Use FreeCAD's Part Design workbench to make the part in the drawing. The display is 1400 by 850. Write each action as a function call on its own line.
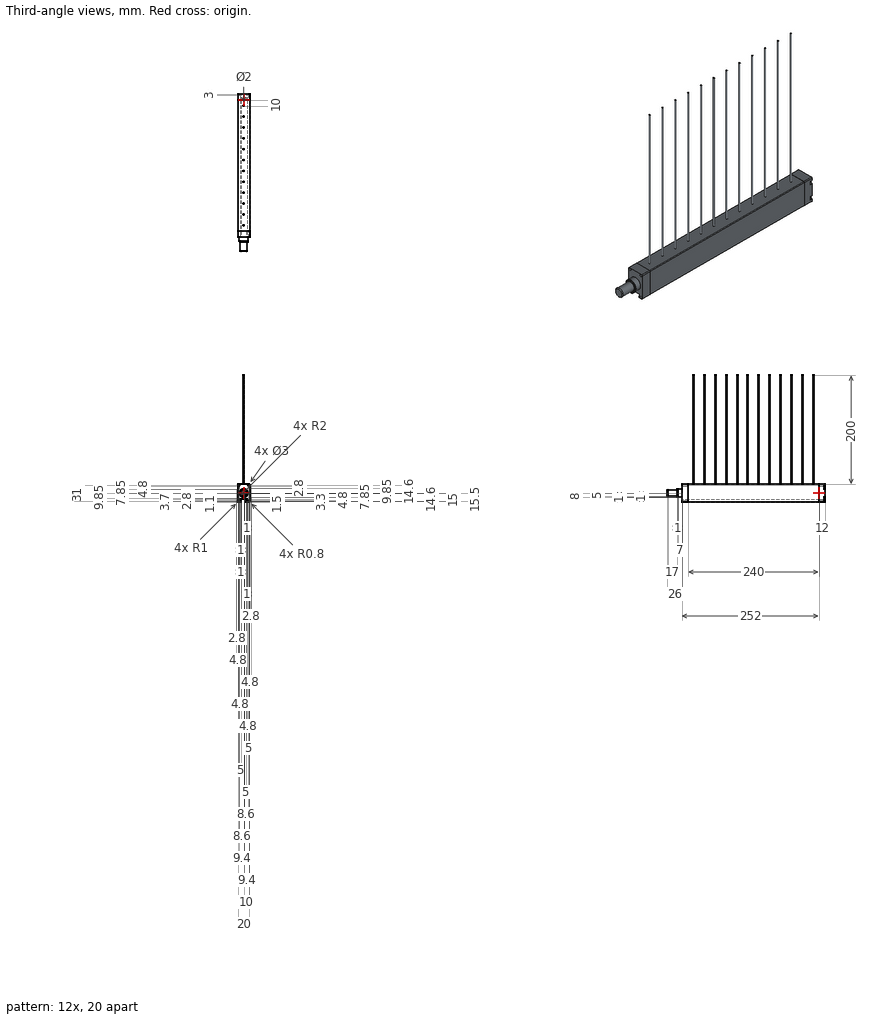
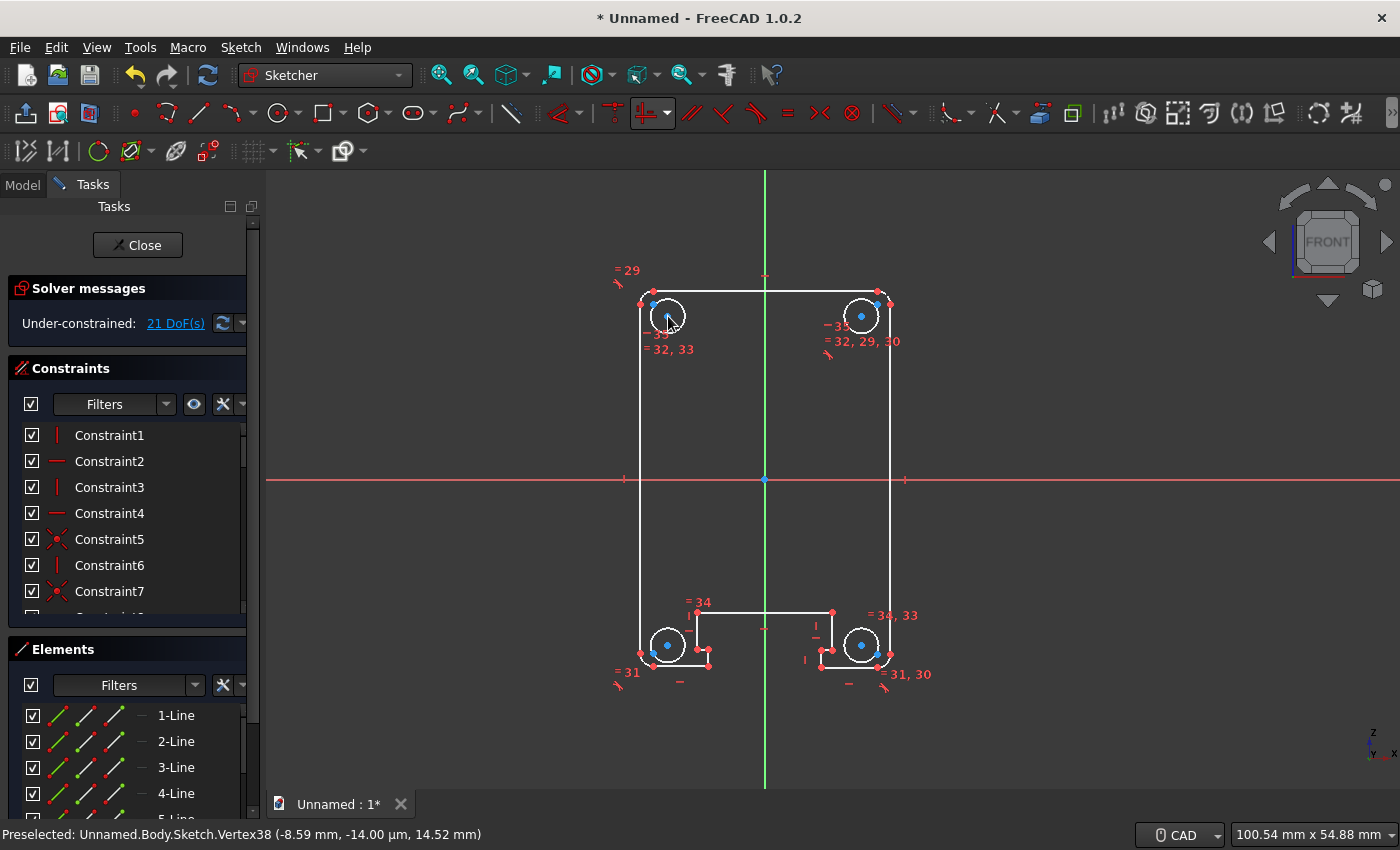
click(558, 114)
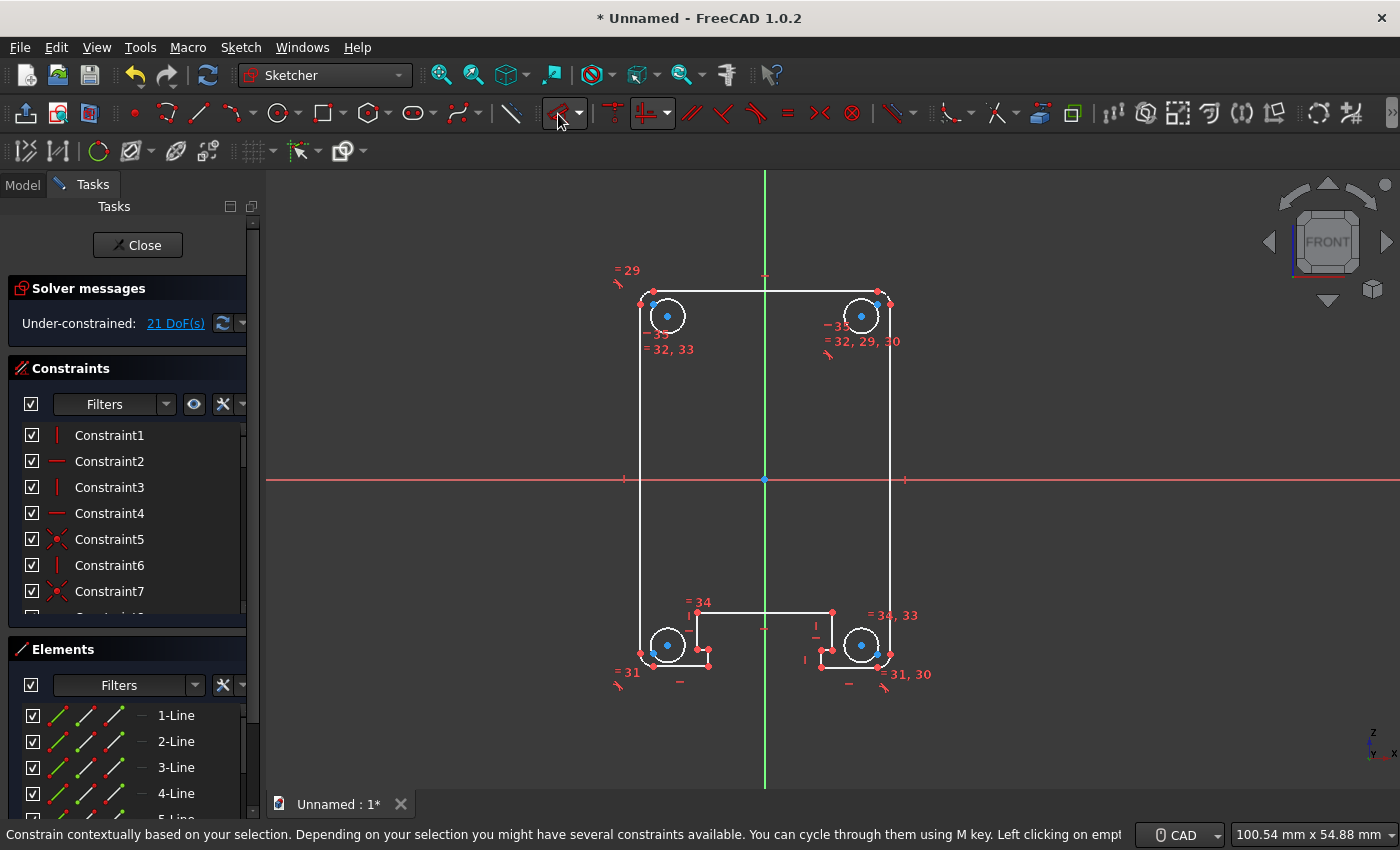
scroll(644, 295, up, 7)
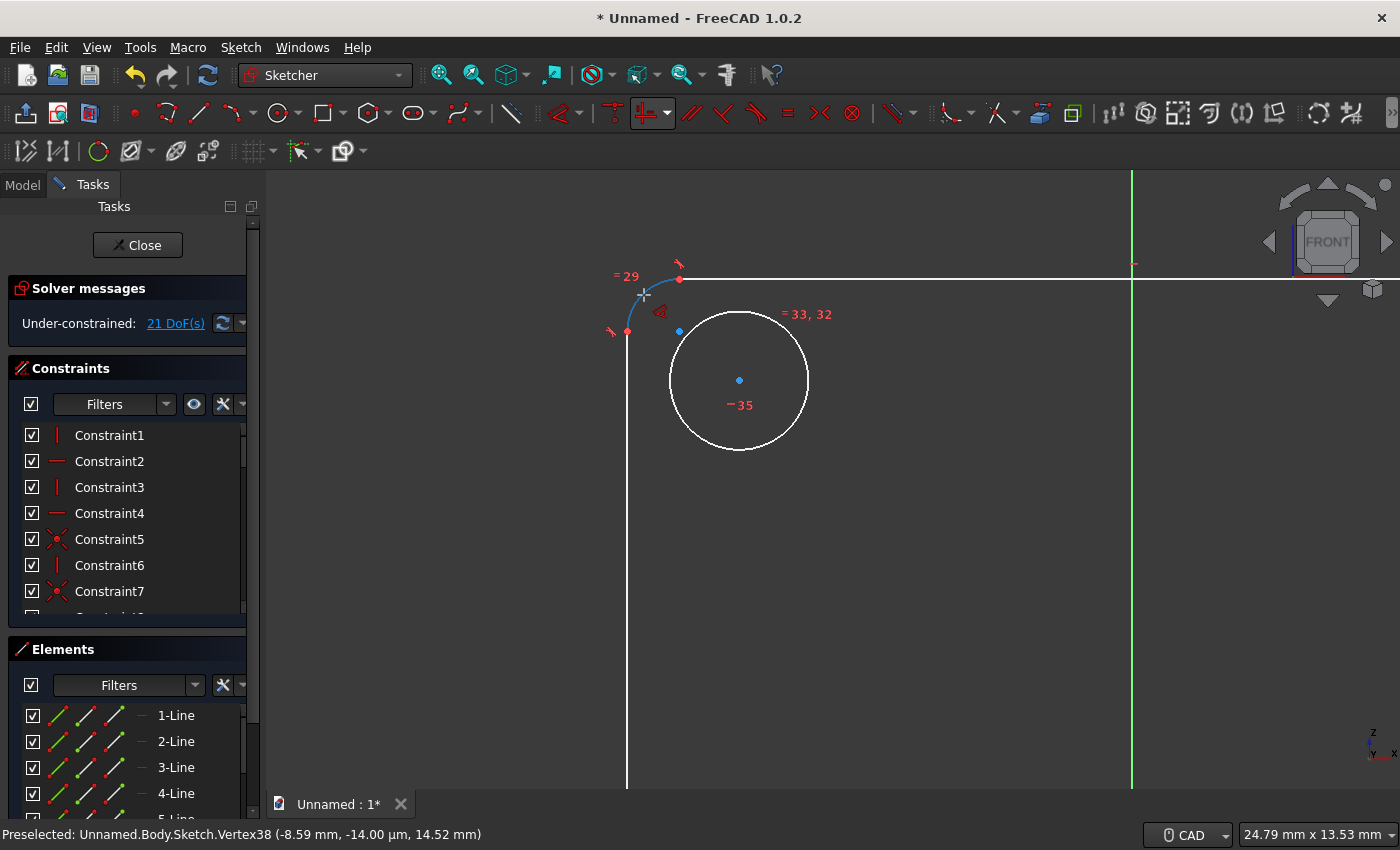
click(643, 294)
click(621, 271)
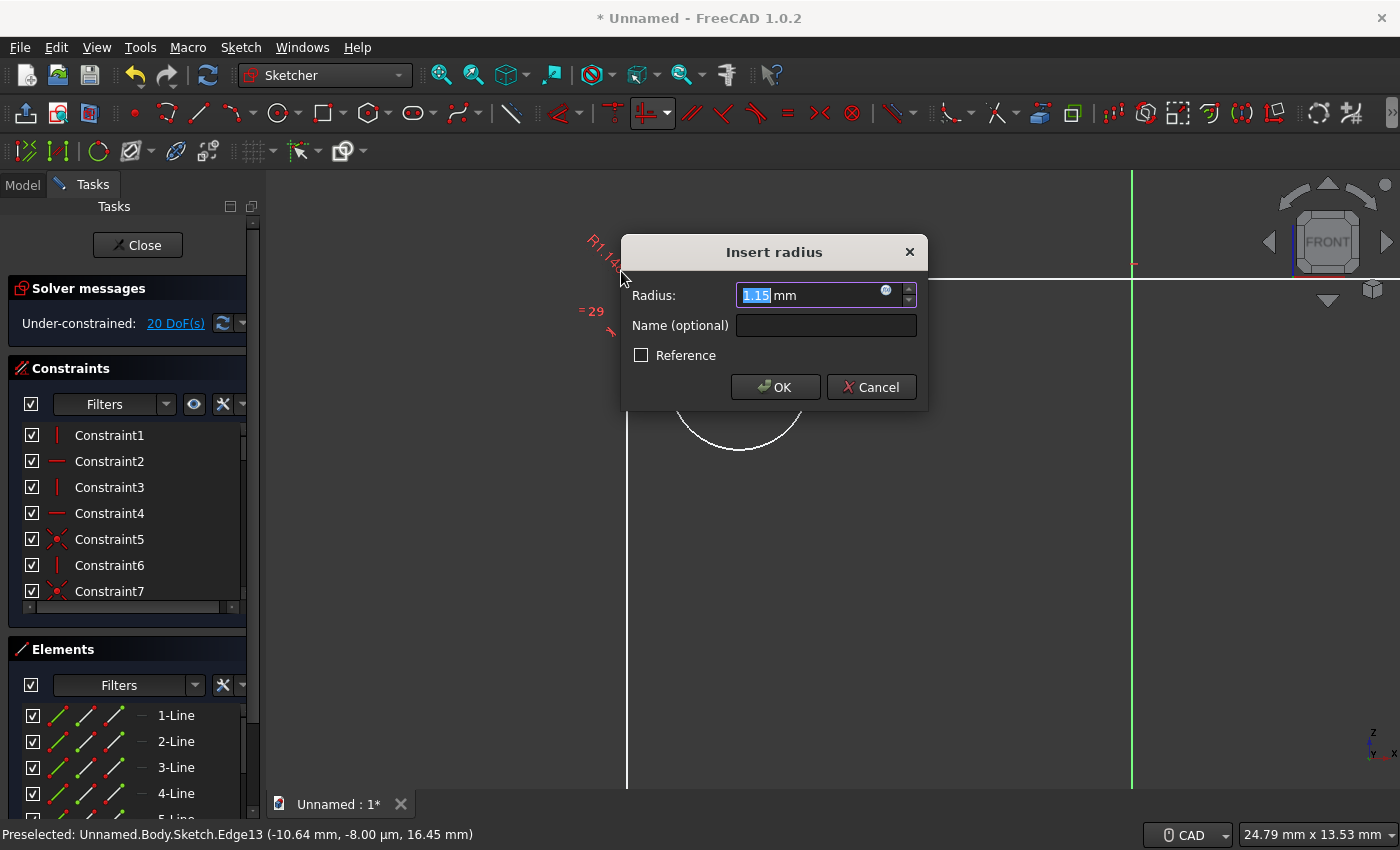
text(1)
key(Return)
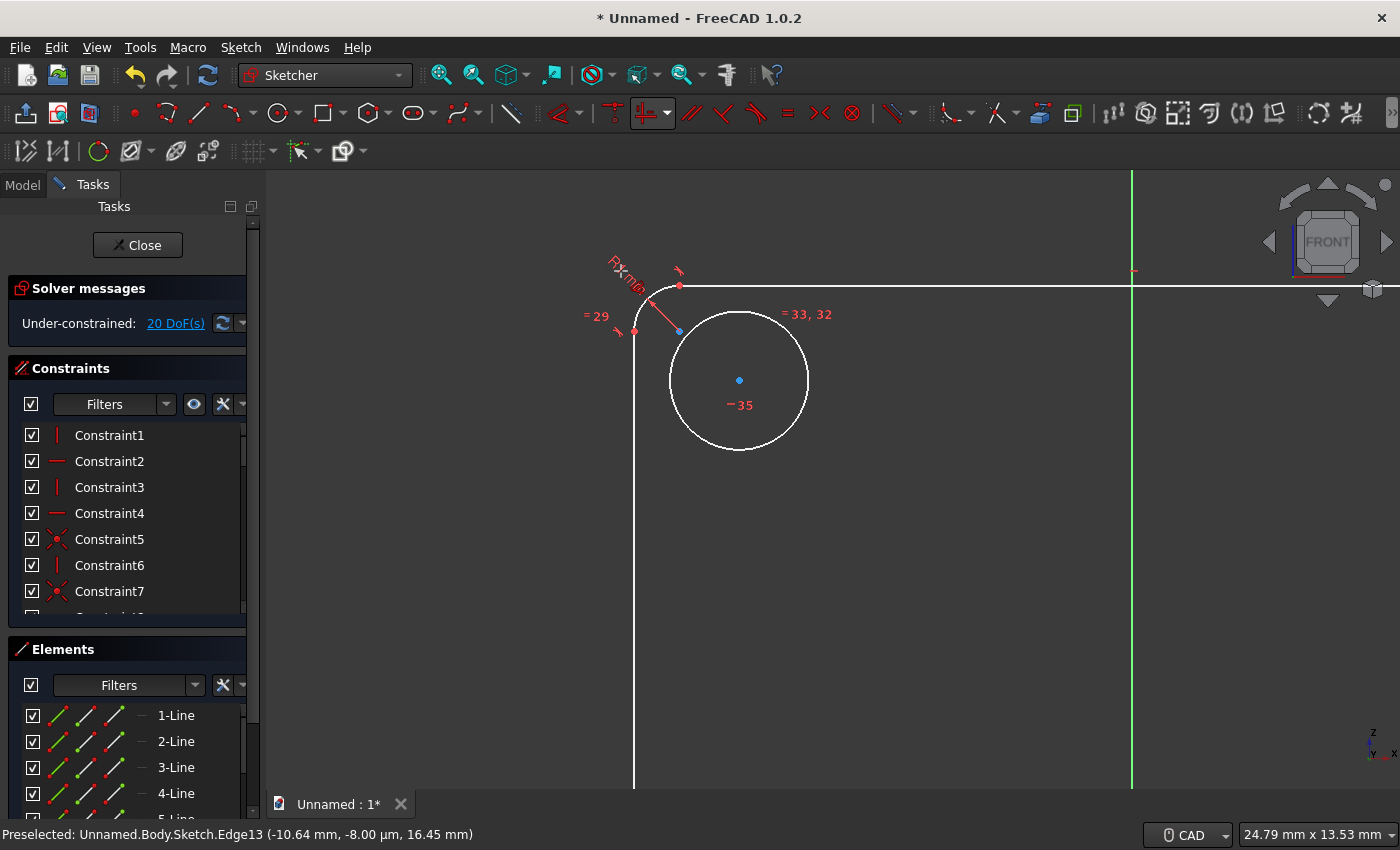
scroll(644, 295, down, 7)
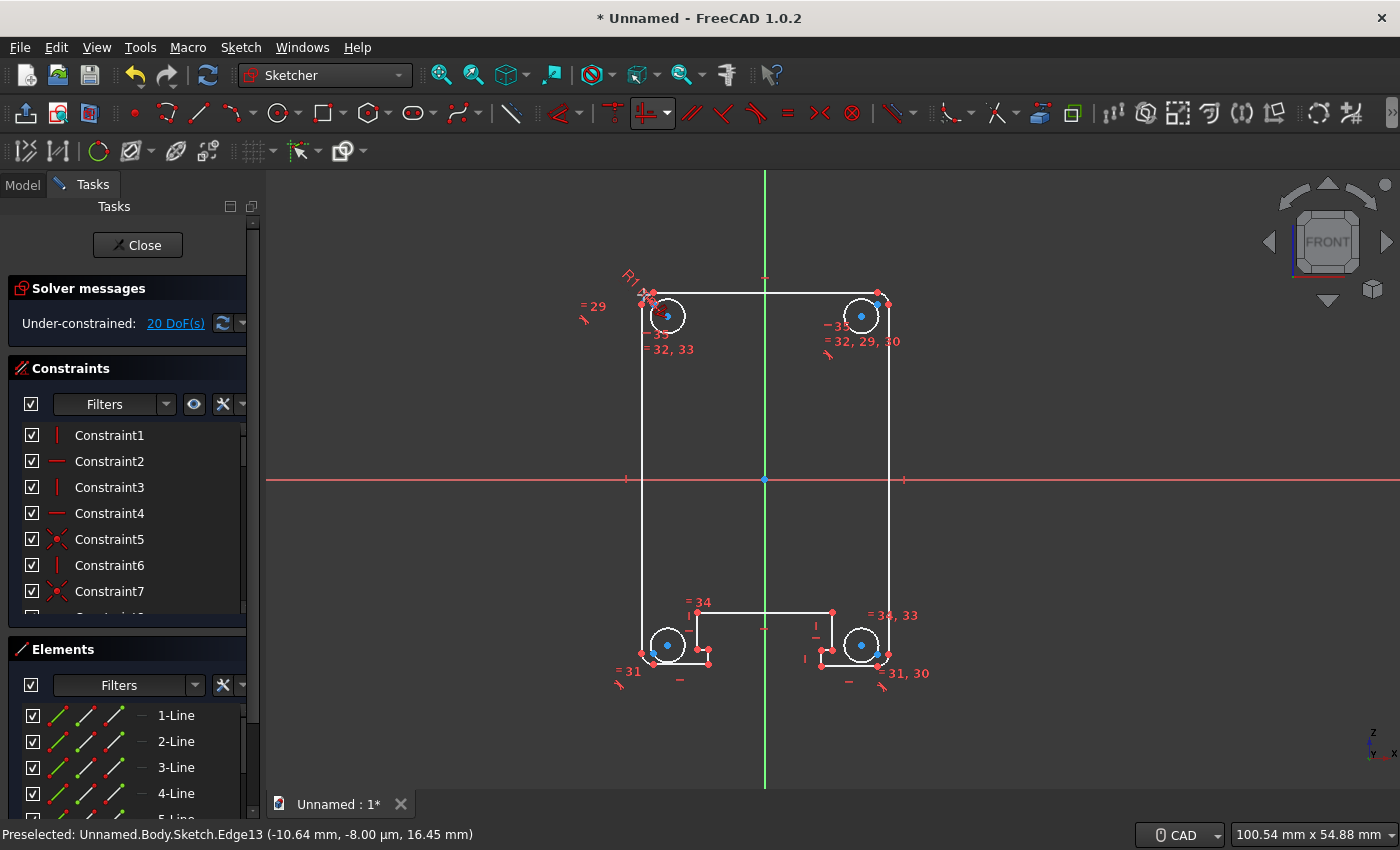
scroll(873, 304, up, 2)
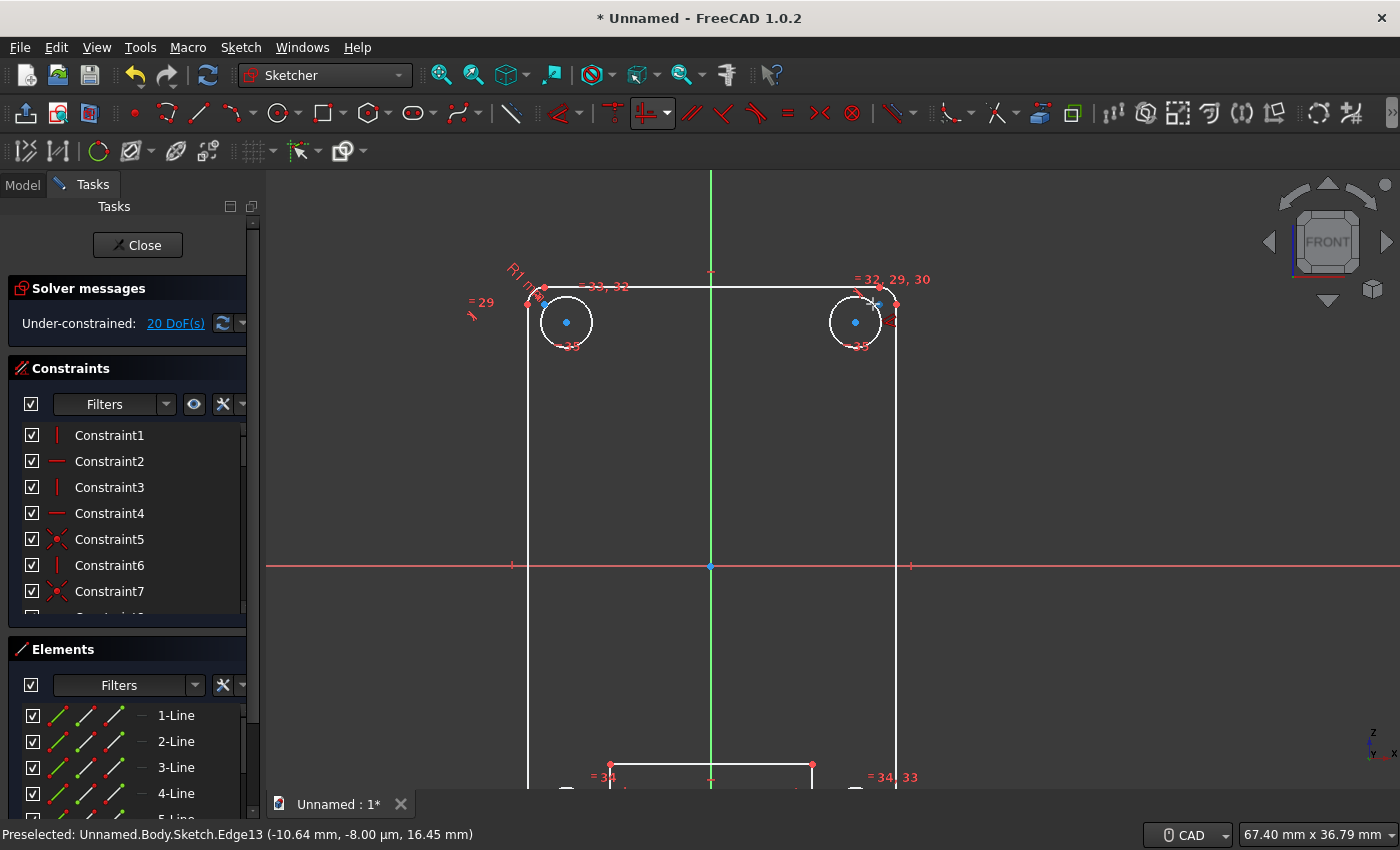
click(873, 304)
click(910, 305)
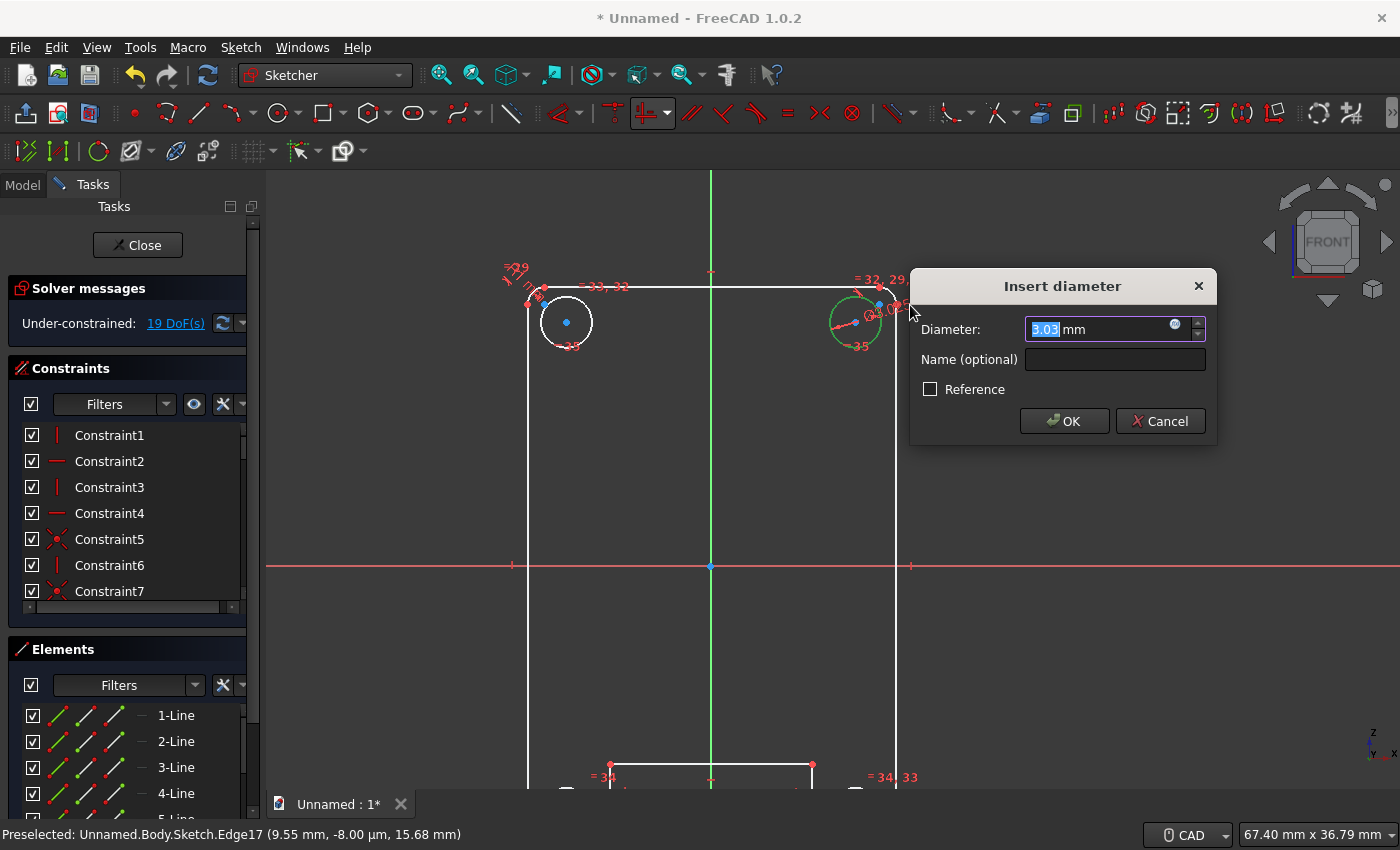
text(3)
key(Return)